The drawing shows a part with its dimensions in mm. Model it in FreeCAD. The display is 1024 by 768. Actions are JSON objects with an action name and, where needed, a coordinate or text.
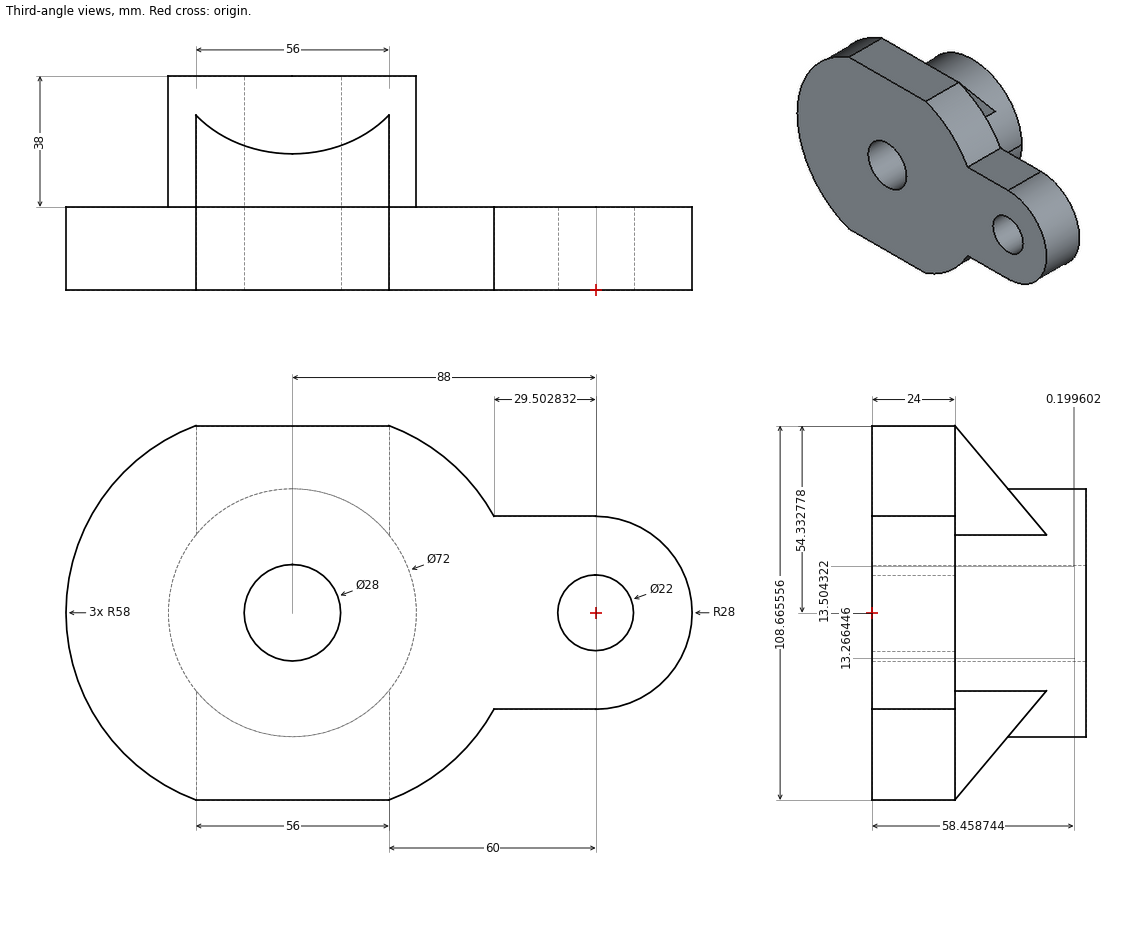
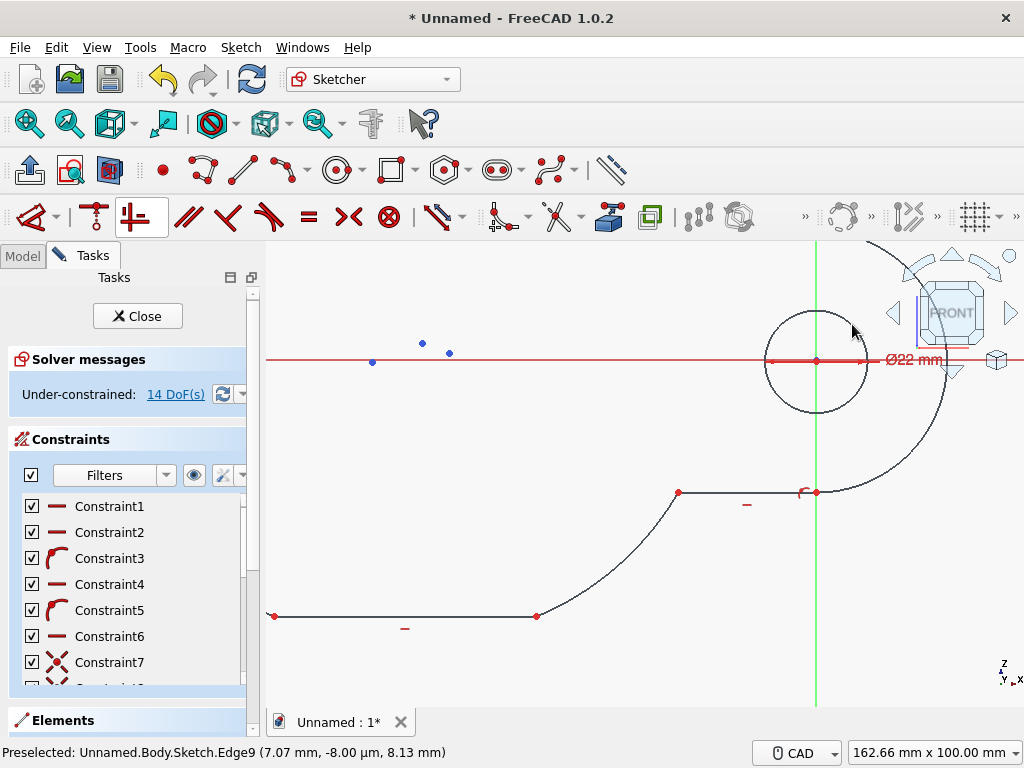
{"action": "scroll", "coordinate": [620, 567], "scroll_direction": "down", "scroll_amount": 4}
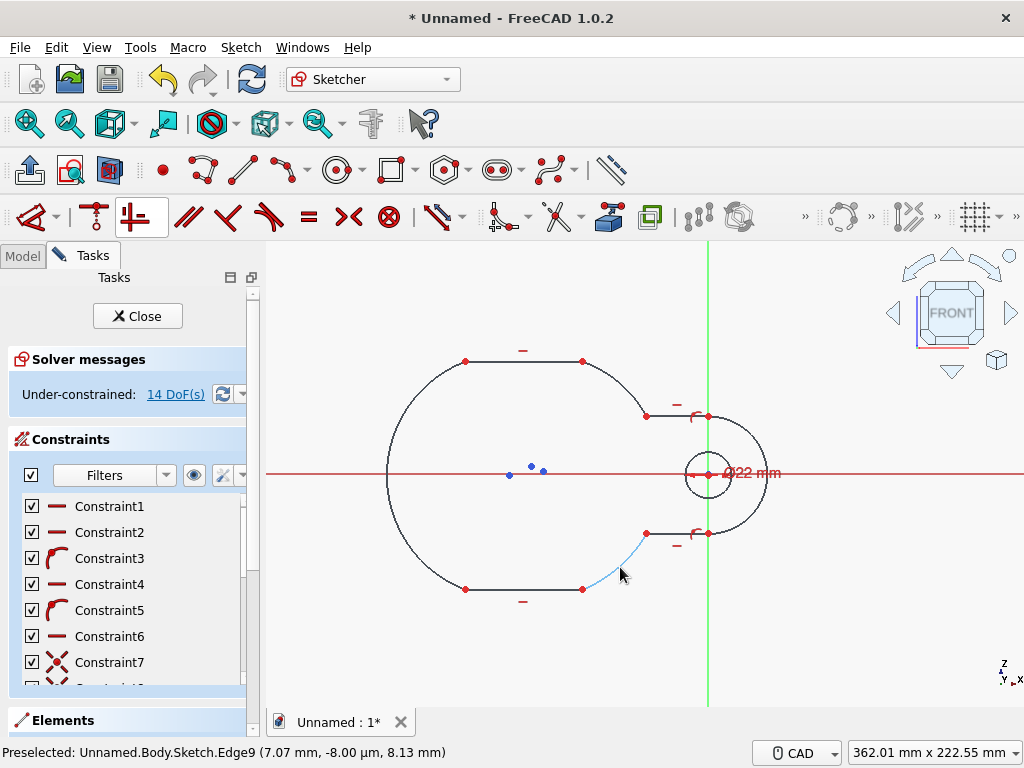
{"action": "left_click", "coordinate": [632, 395]}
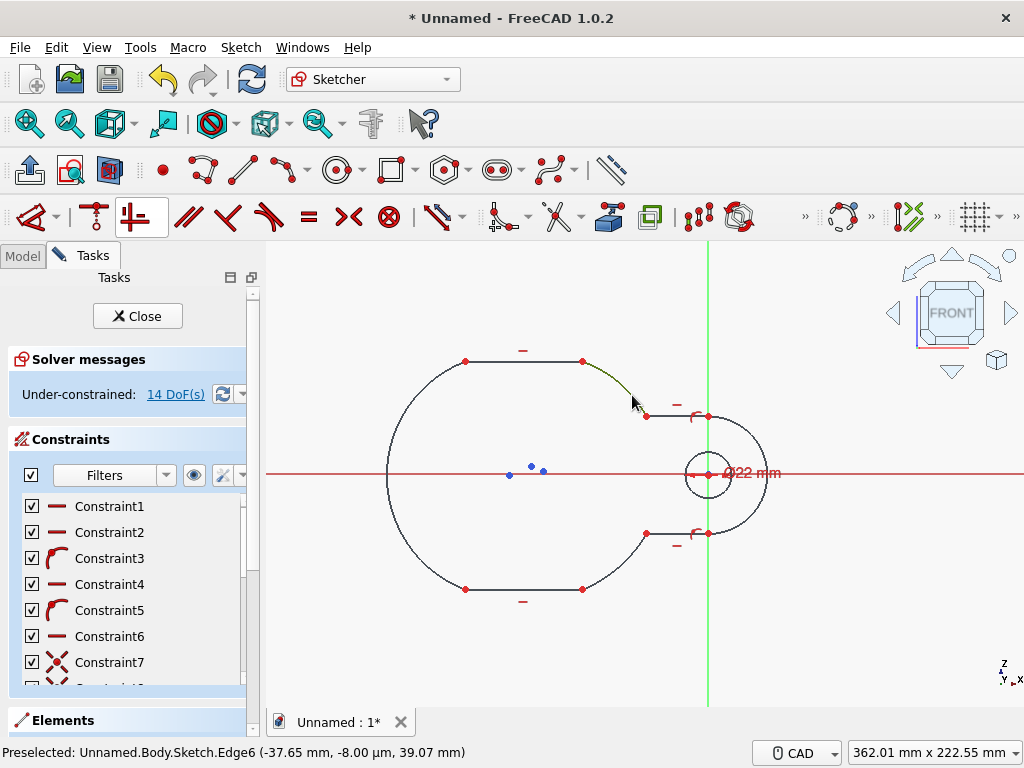
{"action": "left_click", "coordinate": [605, 578]}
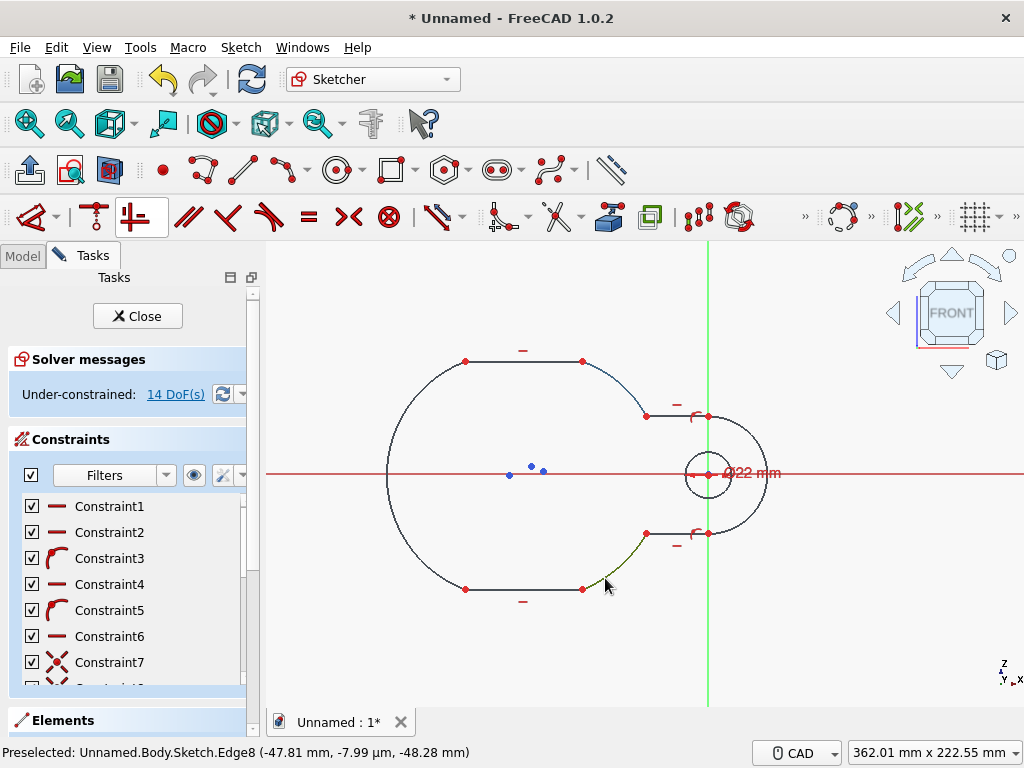
{"action": "left_click", "coordinate": [94, 218]}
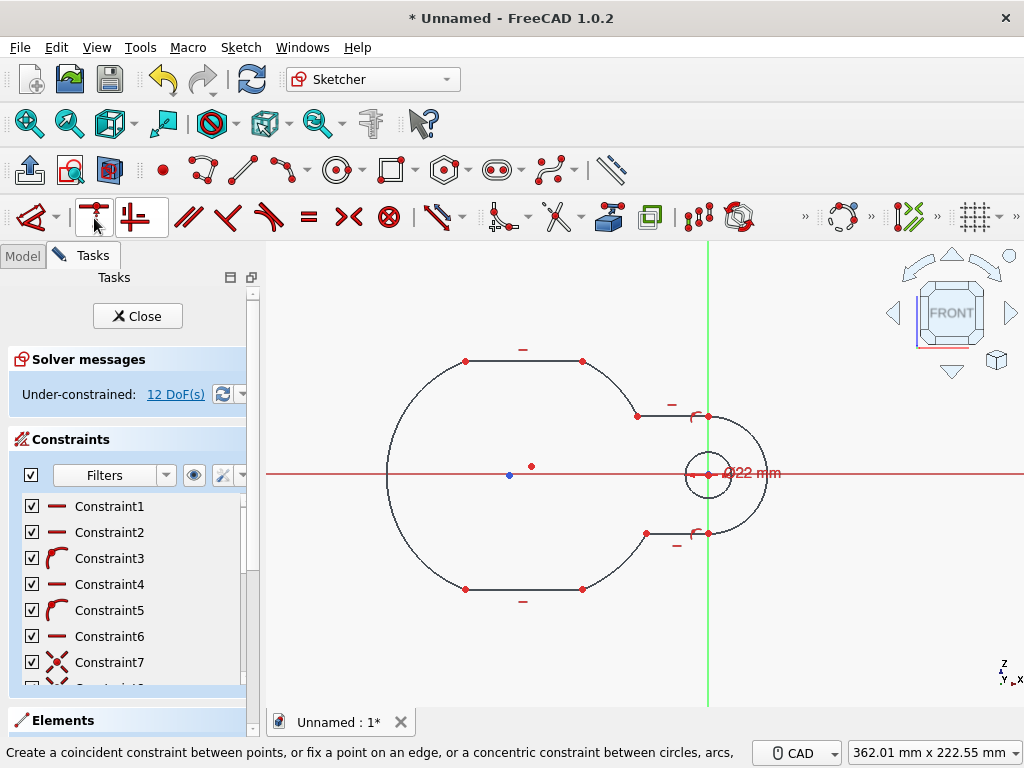
{"action": "scroll", "coordinate": [708, 475], "scroll_direction": "up", "scroll_amount": 3}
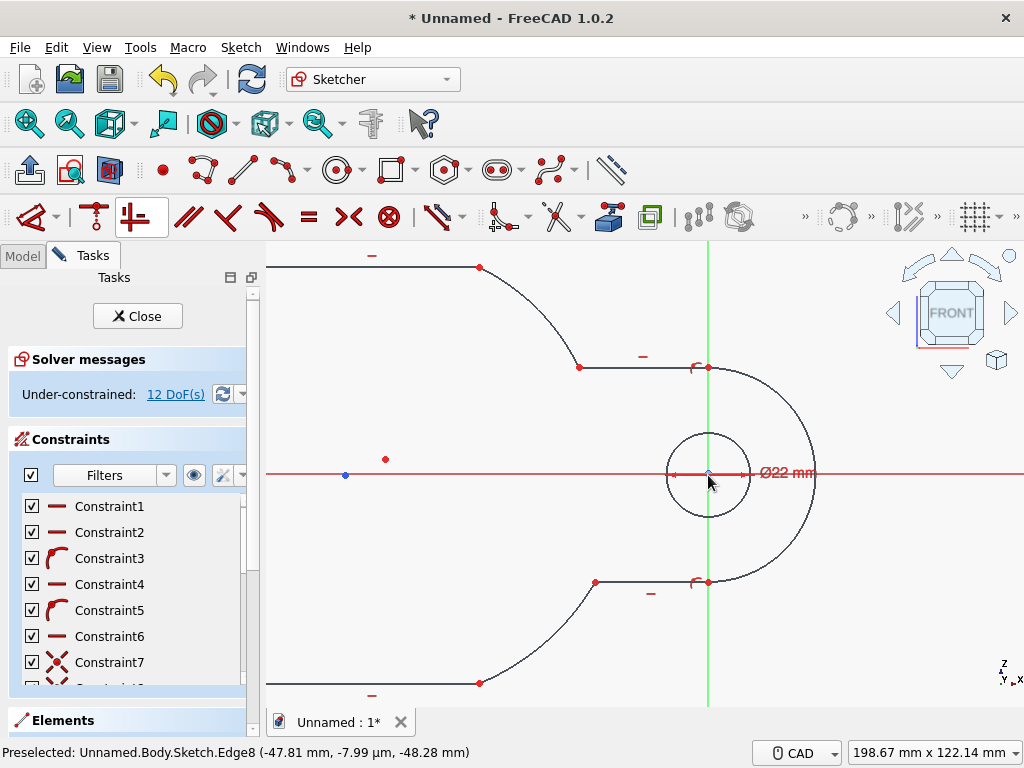
{"action": "left_click_drag", "start_coordinate": [698, 464], "coordinate": [718, 485]}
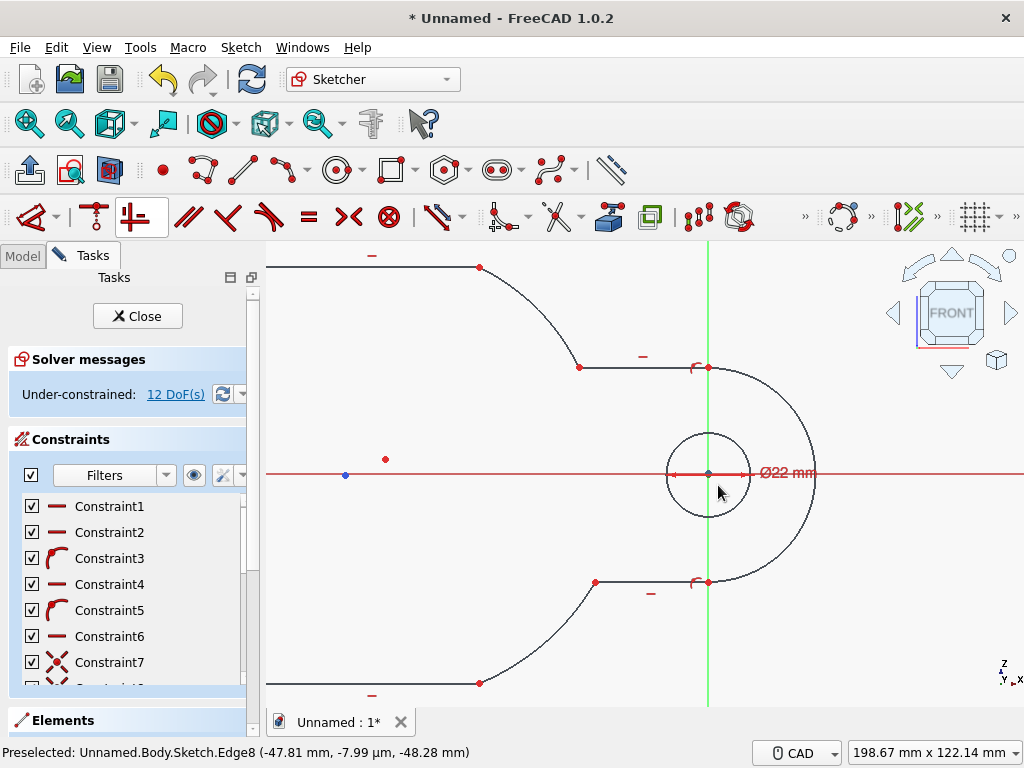
{"action": "left_click", "coordinate": [94, 218]}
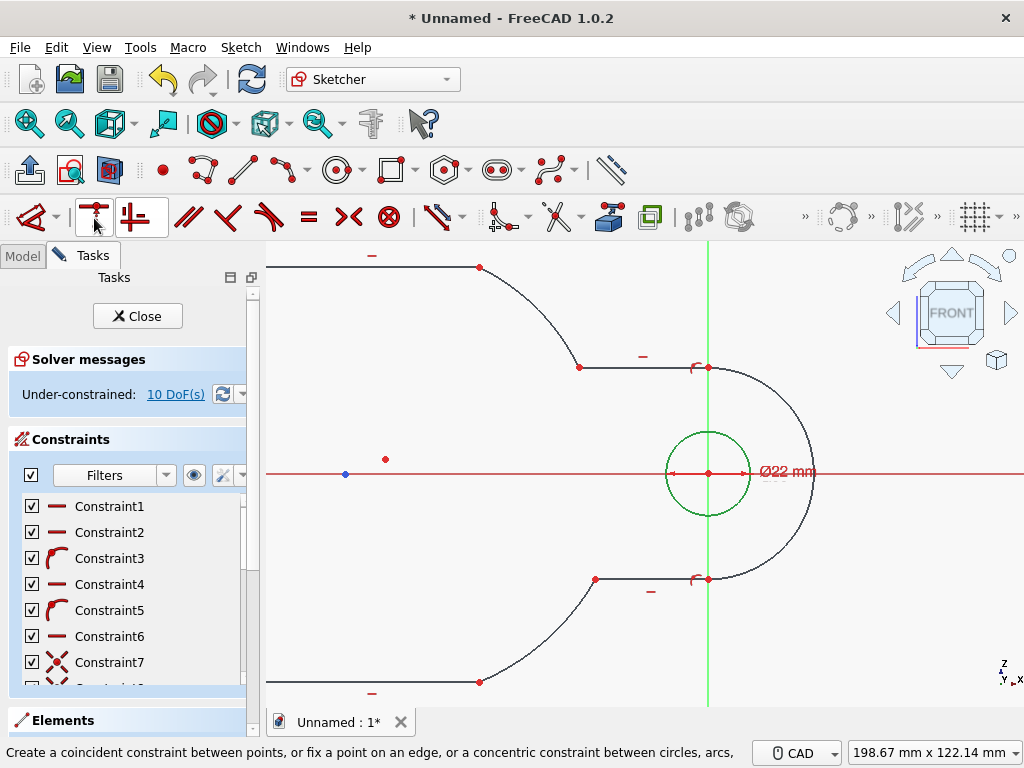
{"action": "scroll", "coordinate": [708, 474], "scroll_direction": "down", "scroll_amount": 3}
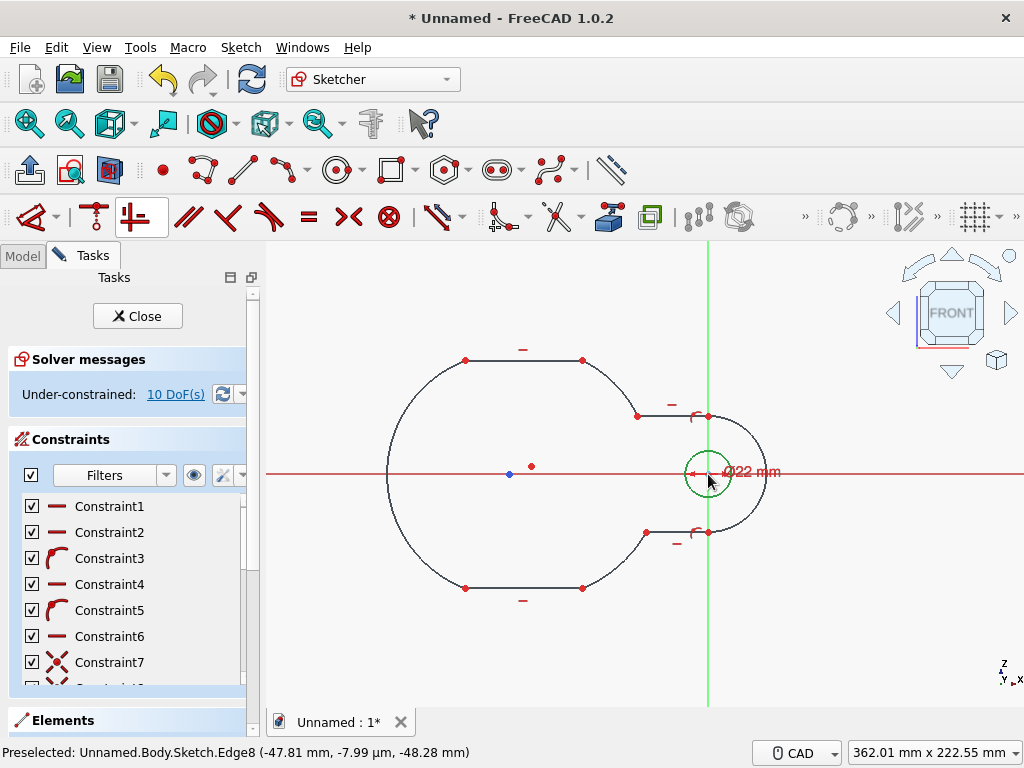
{"action": "left_click", "coordinate": [401, 418]}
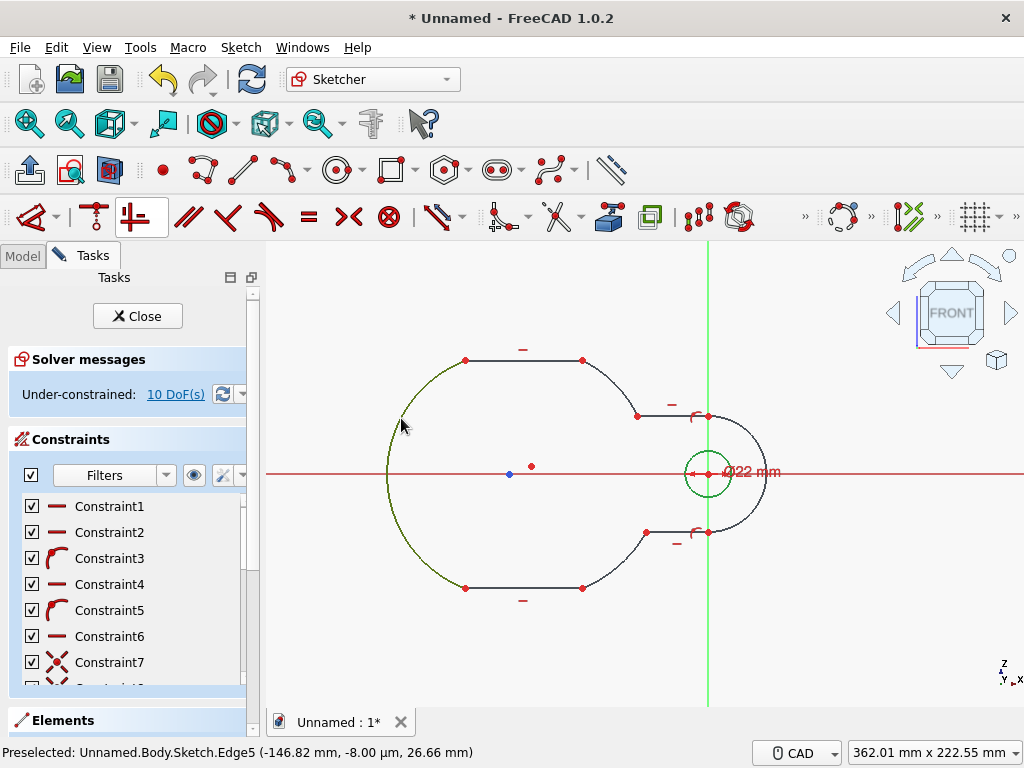
{"action": "left_click", "coordinate": [625, 396]}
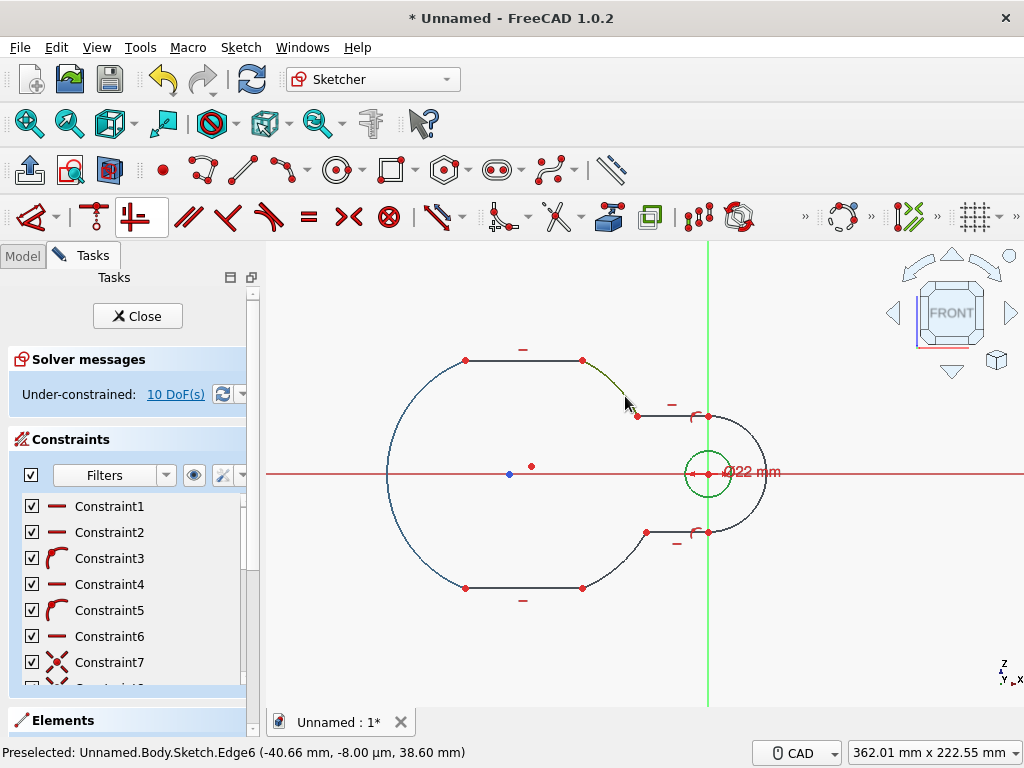
{"action": "left_click", "coordinate": [605, 576]}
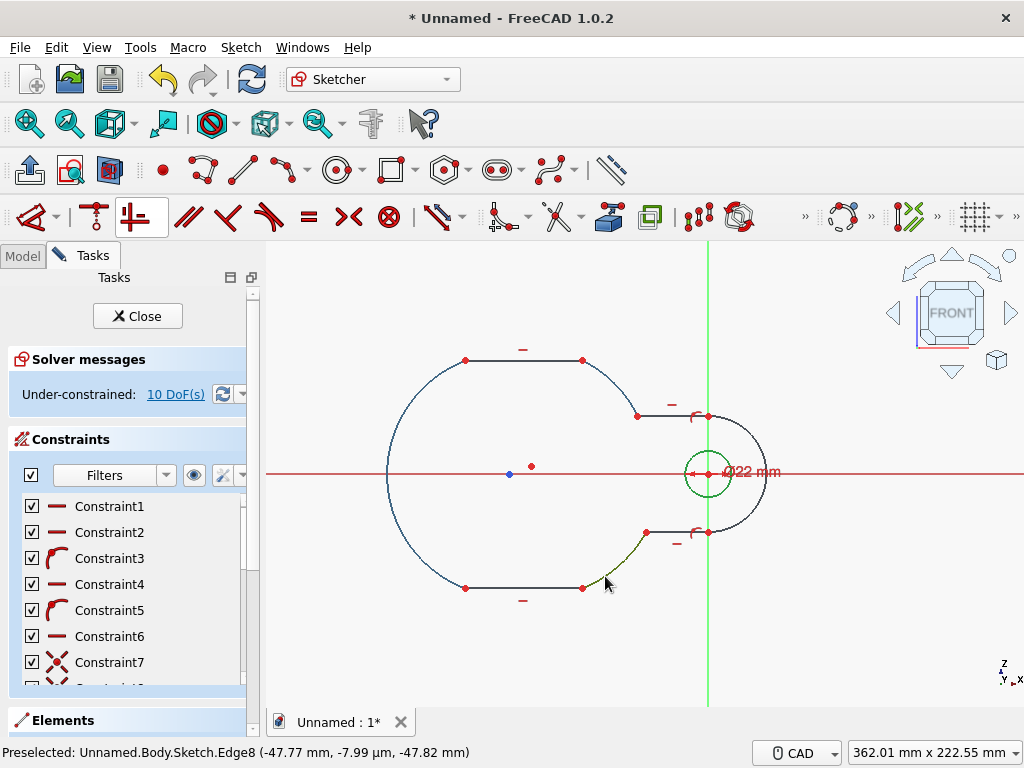
{"action": "left_click", "coordinate": [310, 218]}